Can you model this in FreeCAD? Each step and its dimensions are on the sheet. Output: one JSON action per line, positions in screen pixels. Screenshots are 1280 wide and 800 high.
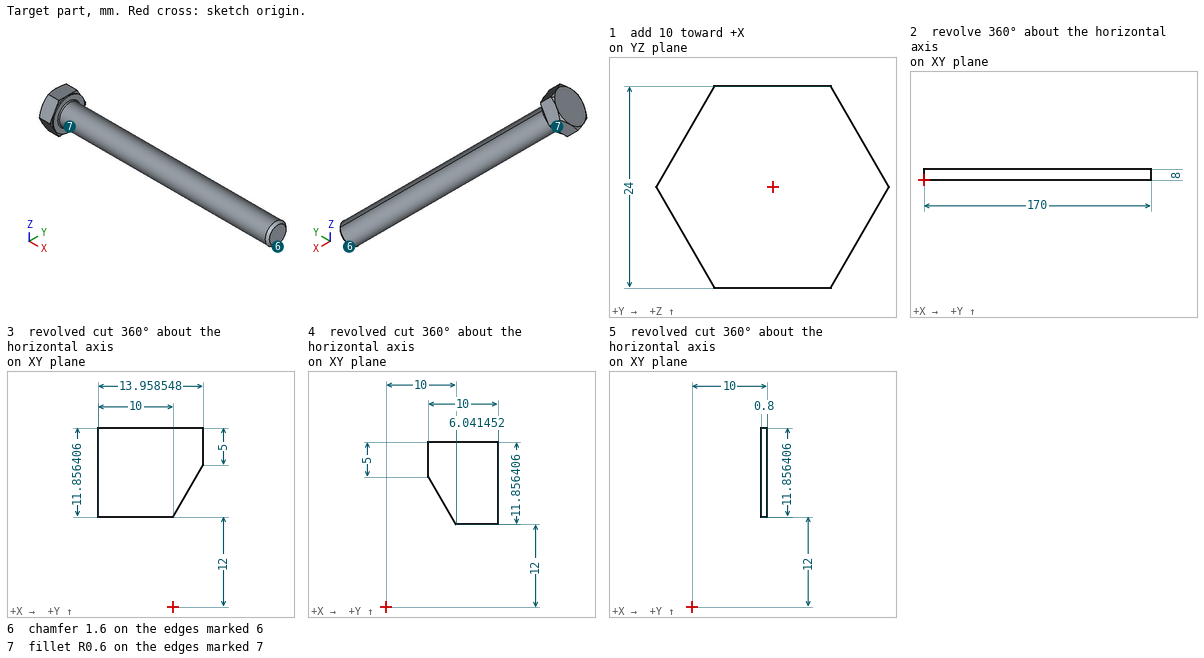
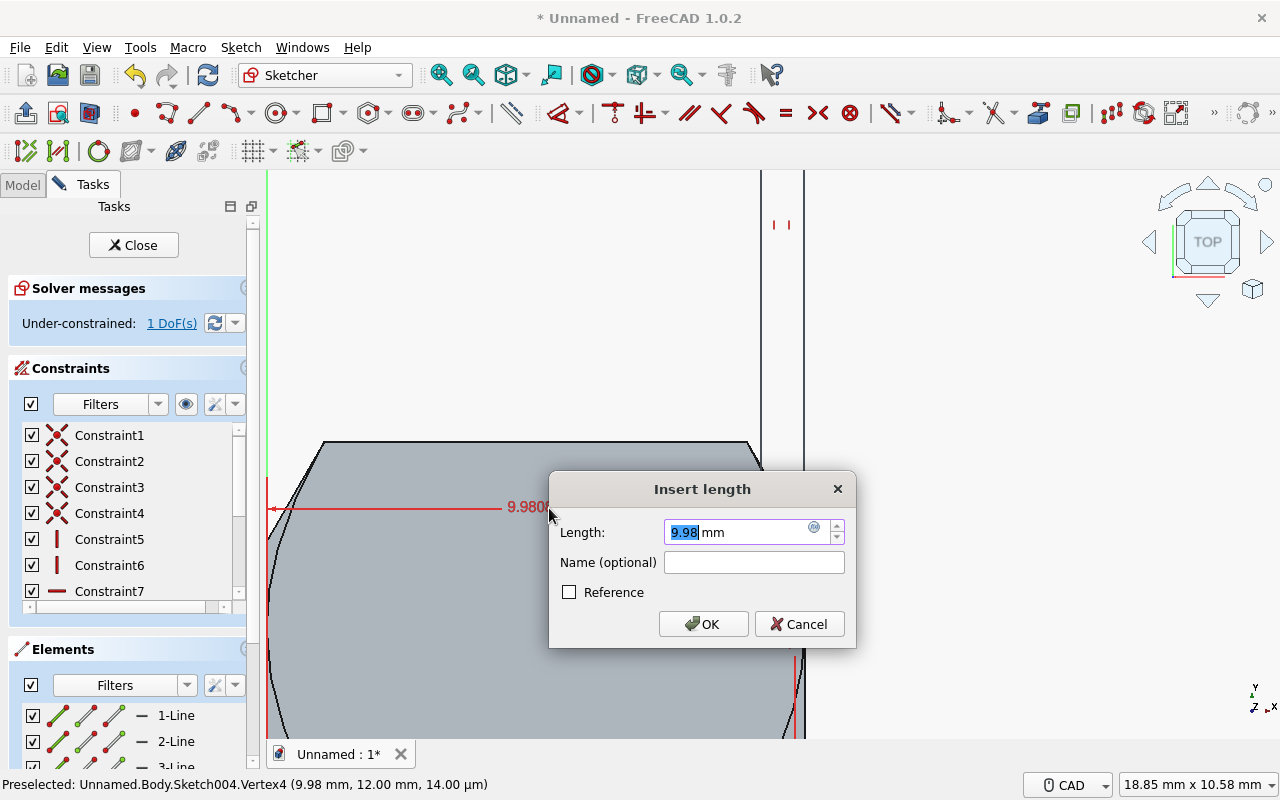
{"action": "type", "text": "10"}
{"action": "key", "text": "Return"}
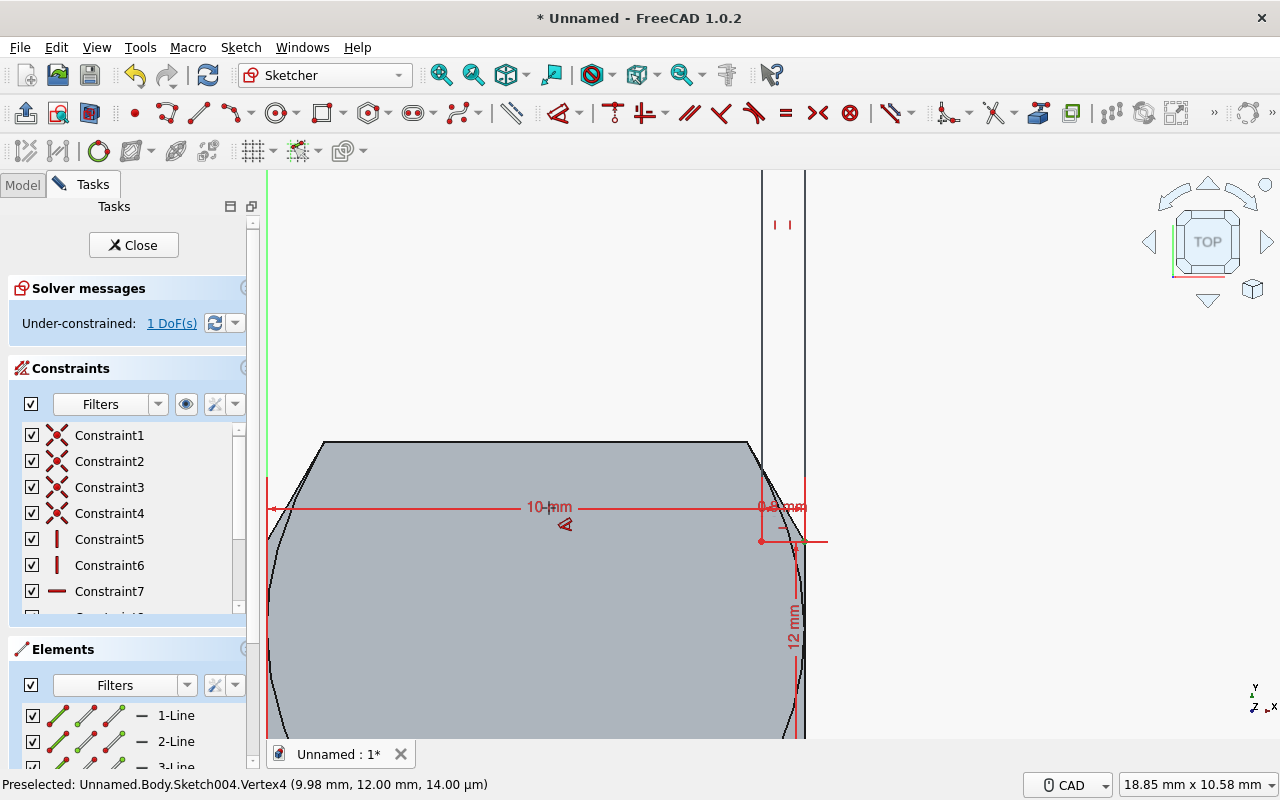
{"action": "left_click", "coordinate": [762, 351]}
{"action": "left_click", "coordinate": [728, 370]}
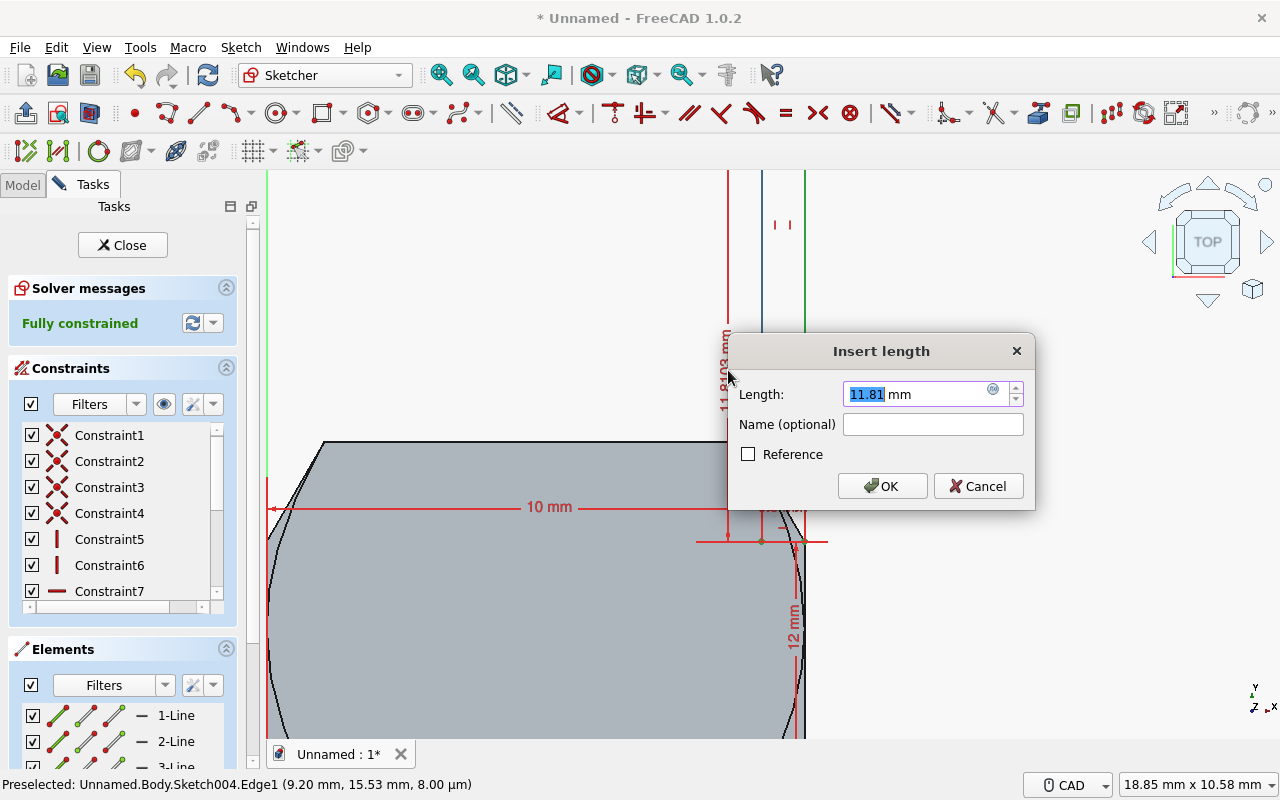
{"action": "type", "text": "11.856406"}
{"action": "key", "text": "Return"}
{"action": "key", "text": "Escape"}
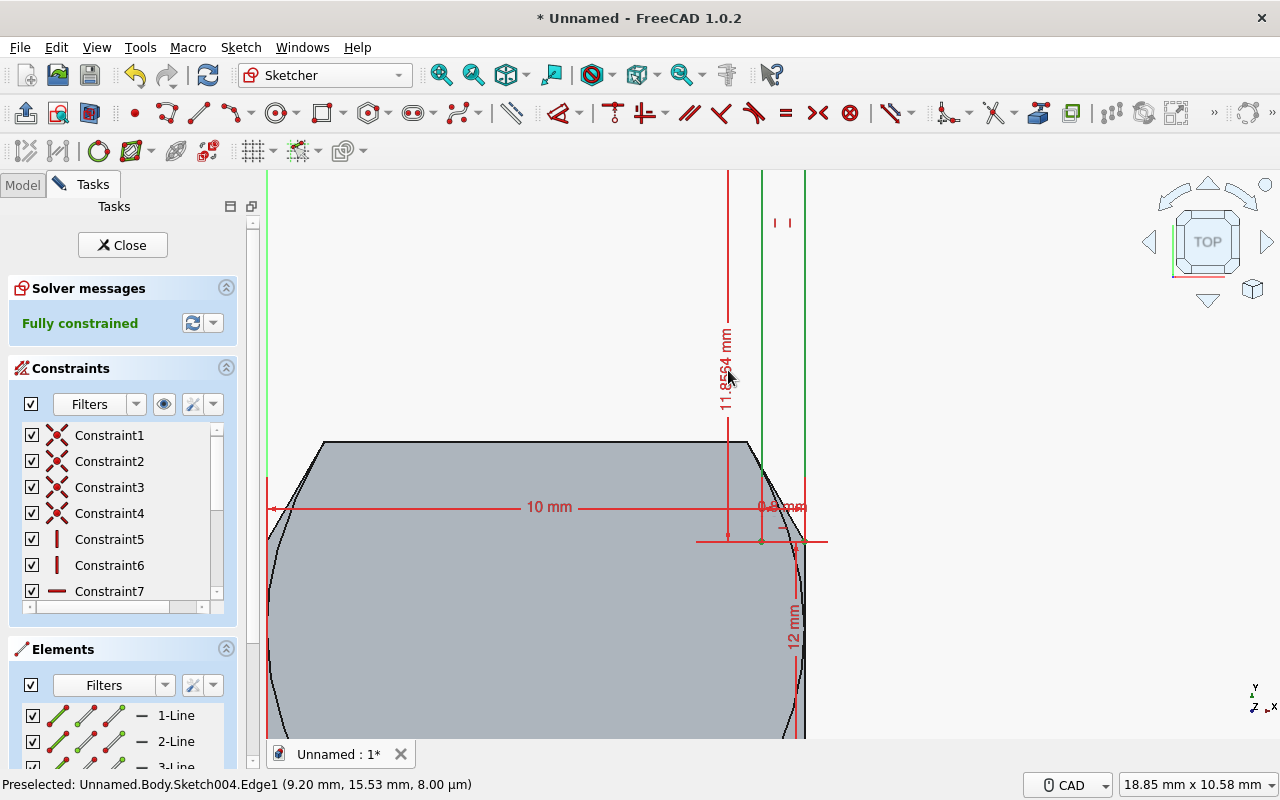
{"action": "left_click", "coordinate": [123, 245]}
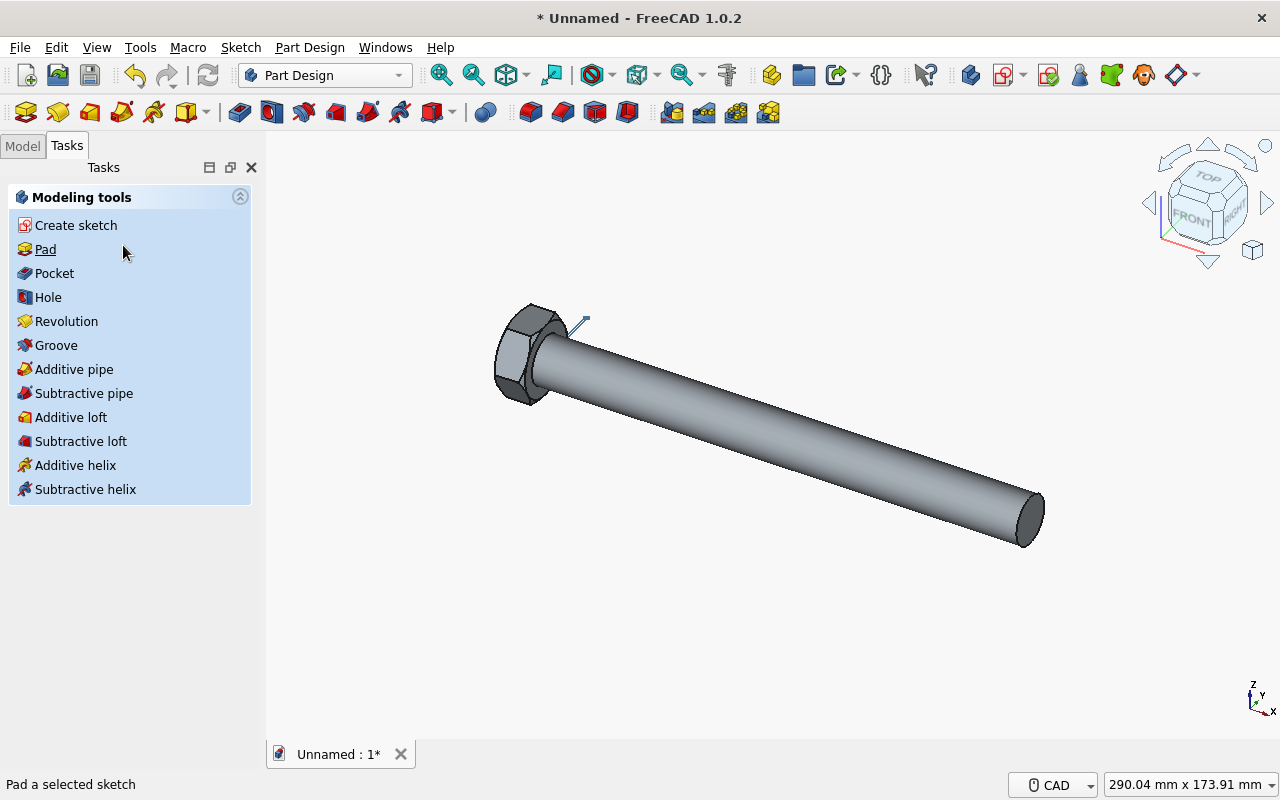
{"action": "left_click", "coordinate": [304, 112]}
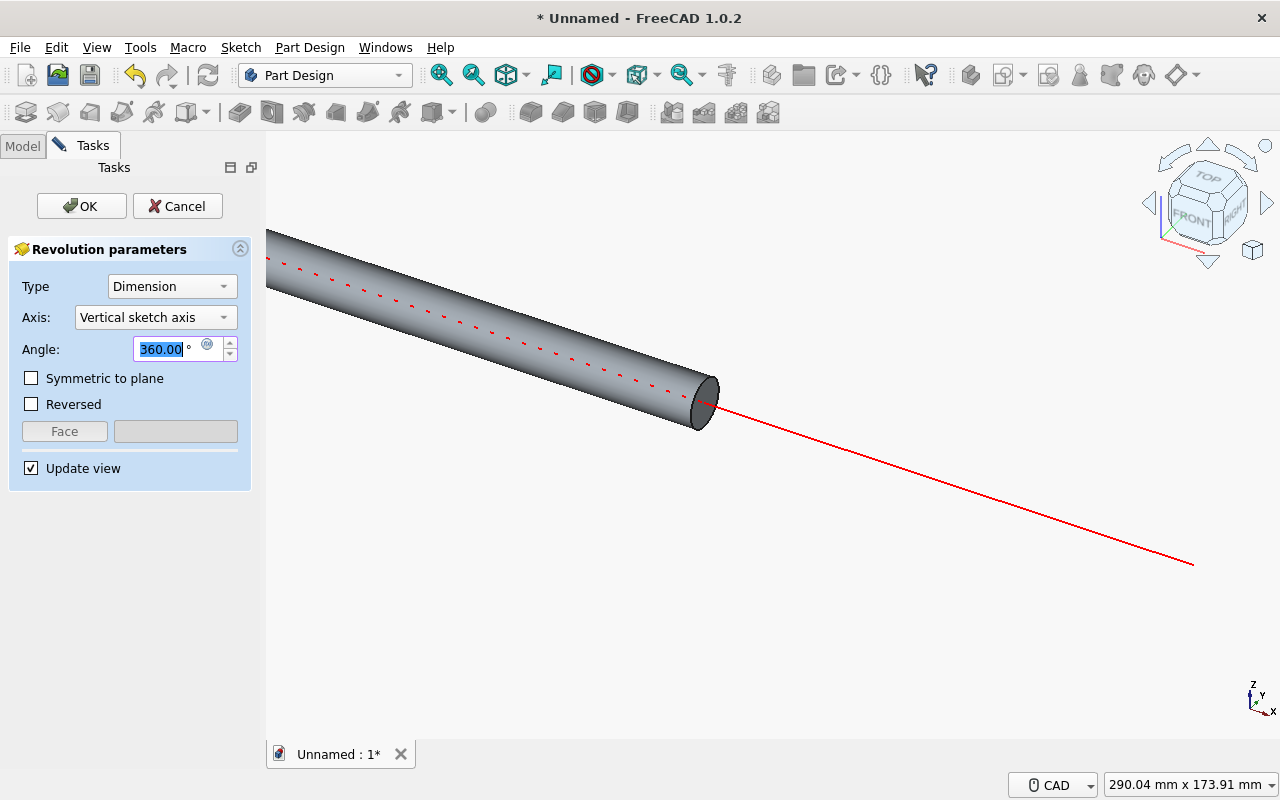
{"action": "left_click", "coordinate": [156, 318]}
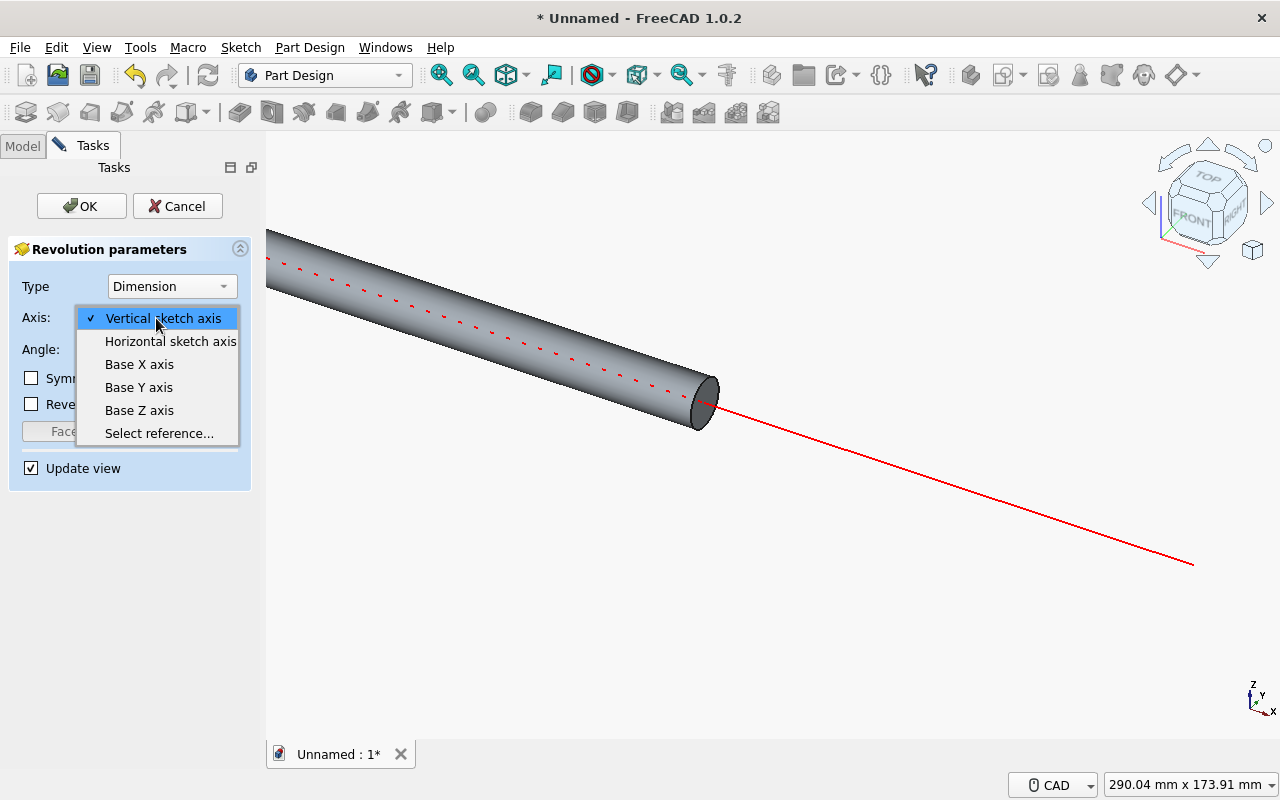
{"action": "left_click", "coordinate": [156, 342]}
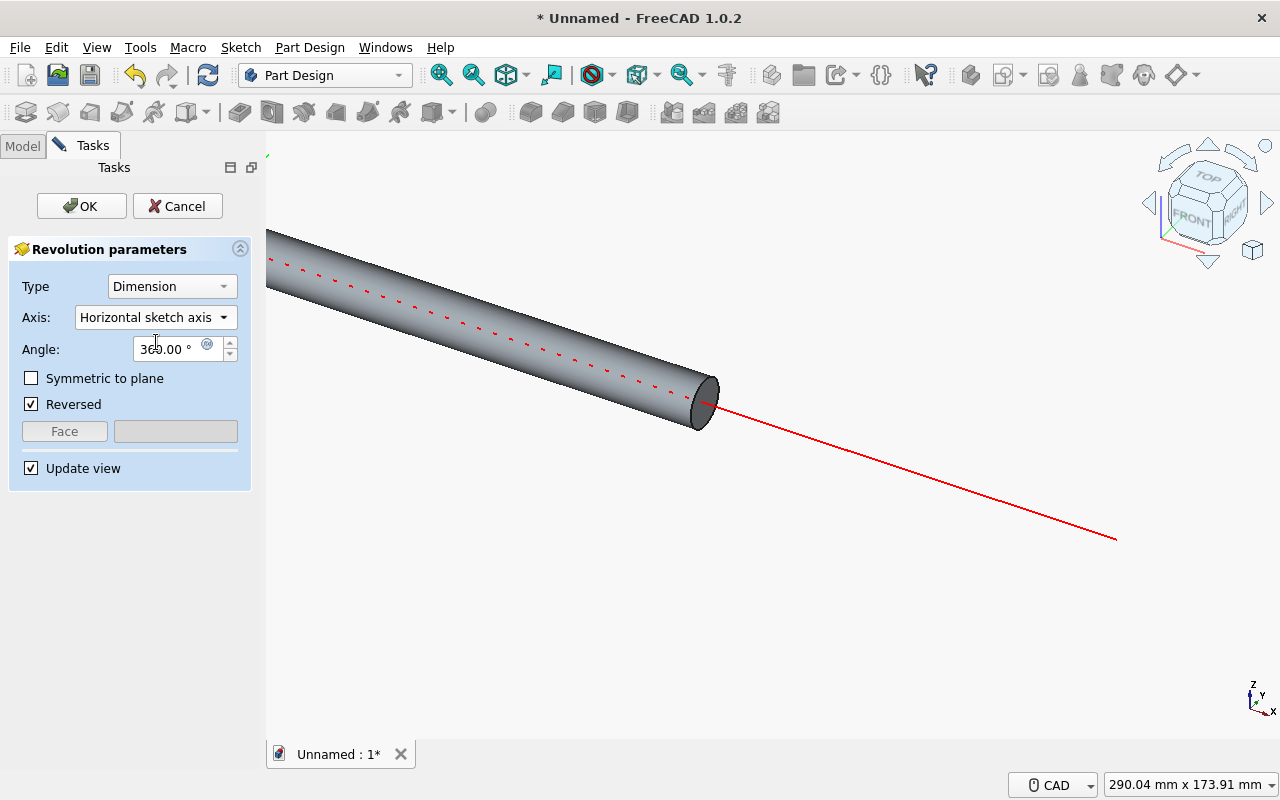
{"action": "left_click", "coordinate": [82, 206]}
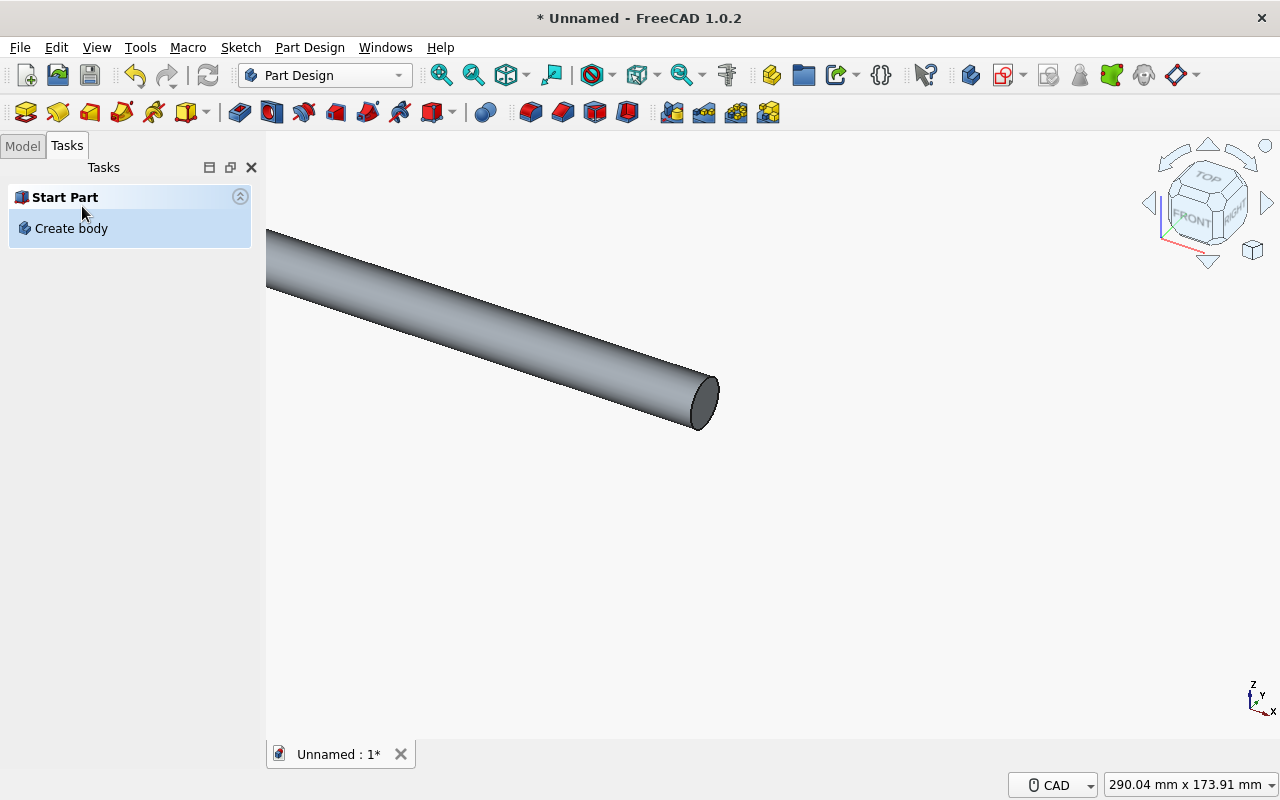
{"action": "left_click", "coordinate": [442, 76]}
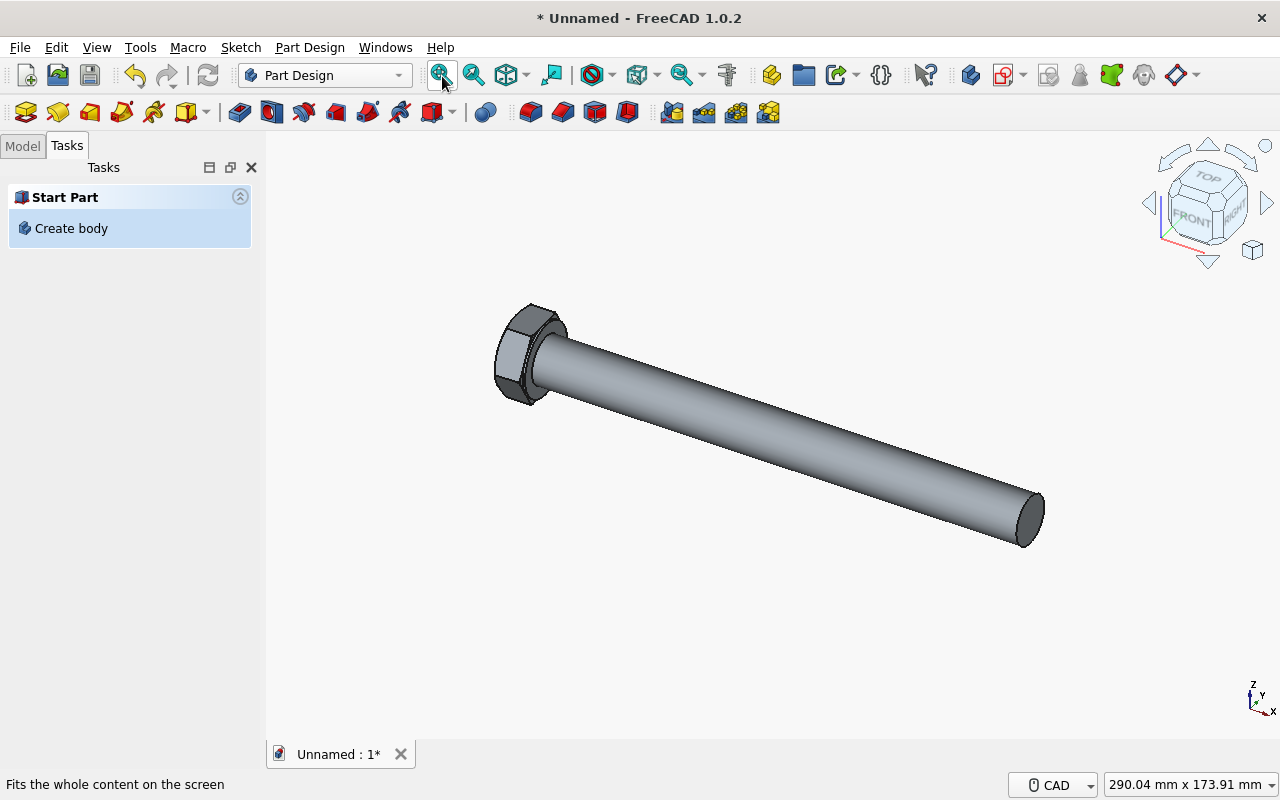
{"action": "left_click", "coordinate": [1016, 533]}